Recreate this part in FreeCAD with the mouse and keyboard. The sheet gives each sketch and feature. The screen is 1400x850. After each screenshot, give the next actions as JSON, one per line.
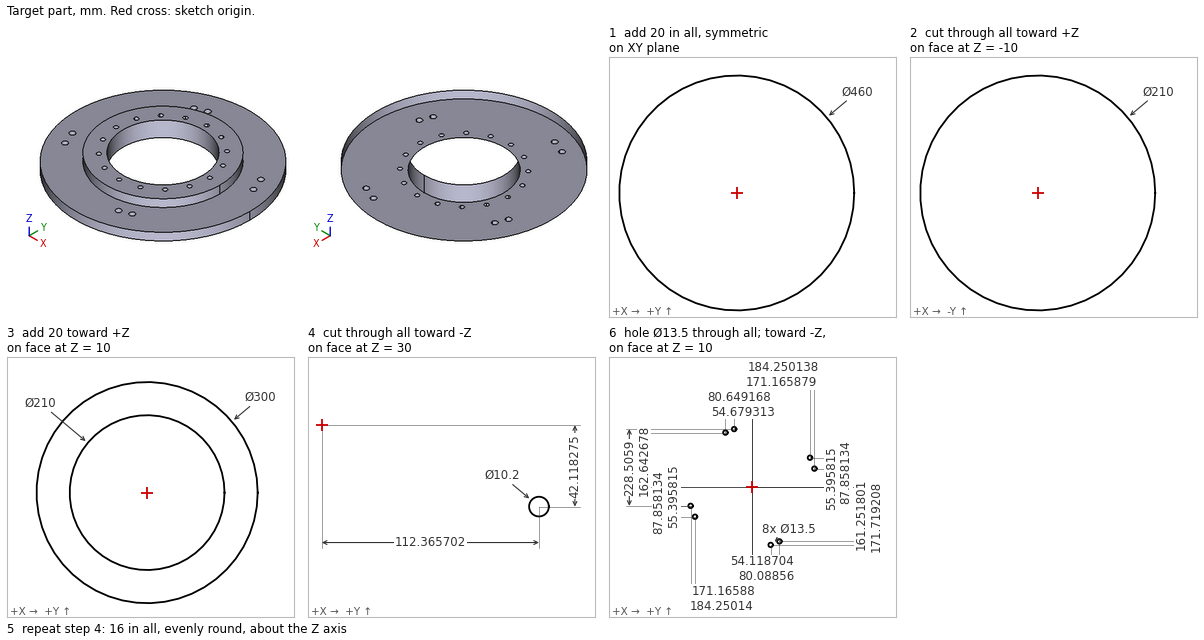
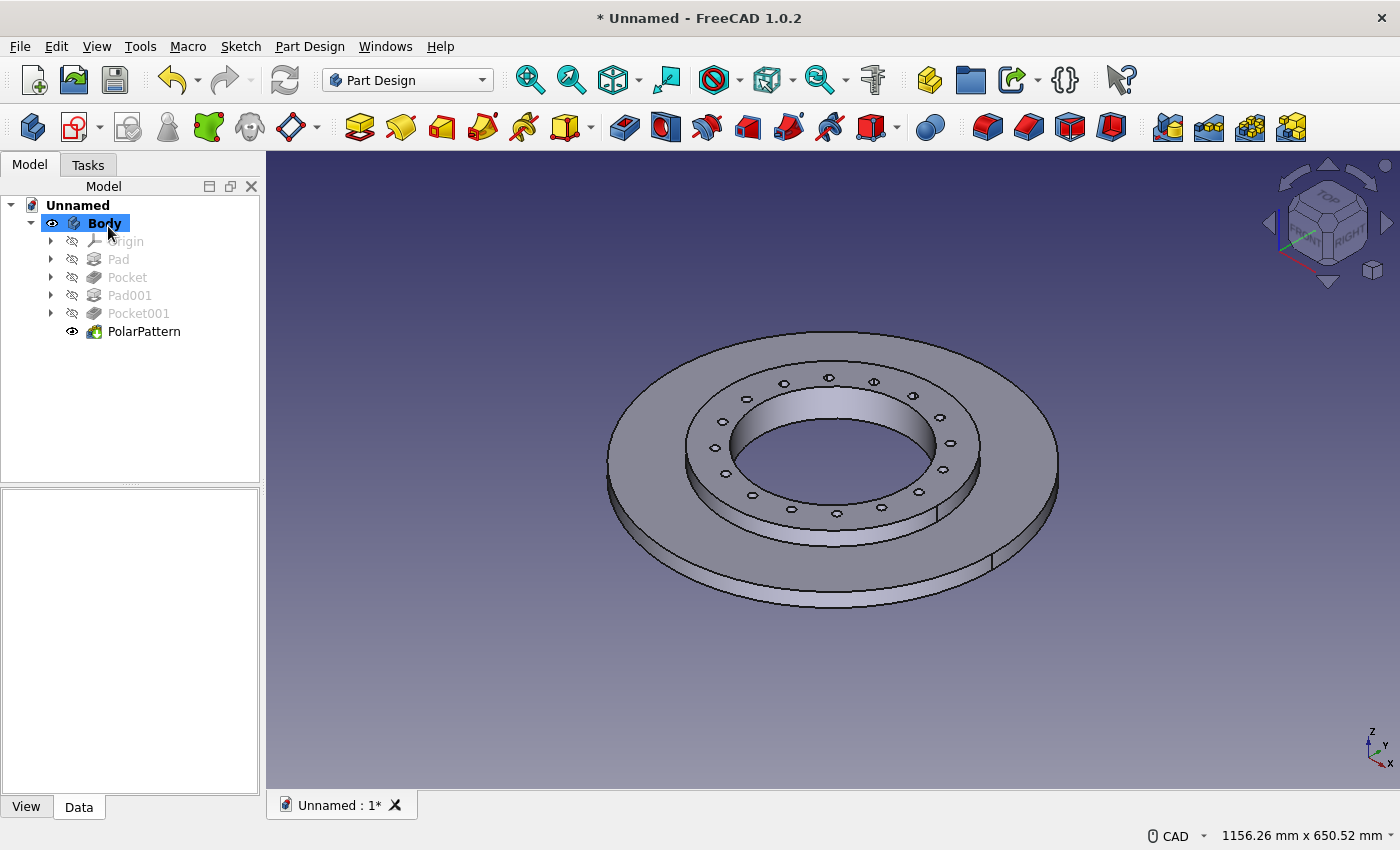
{"action": "left_click", "coordinate": [1015, 461]}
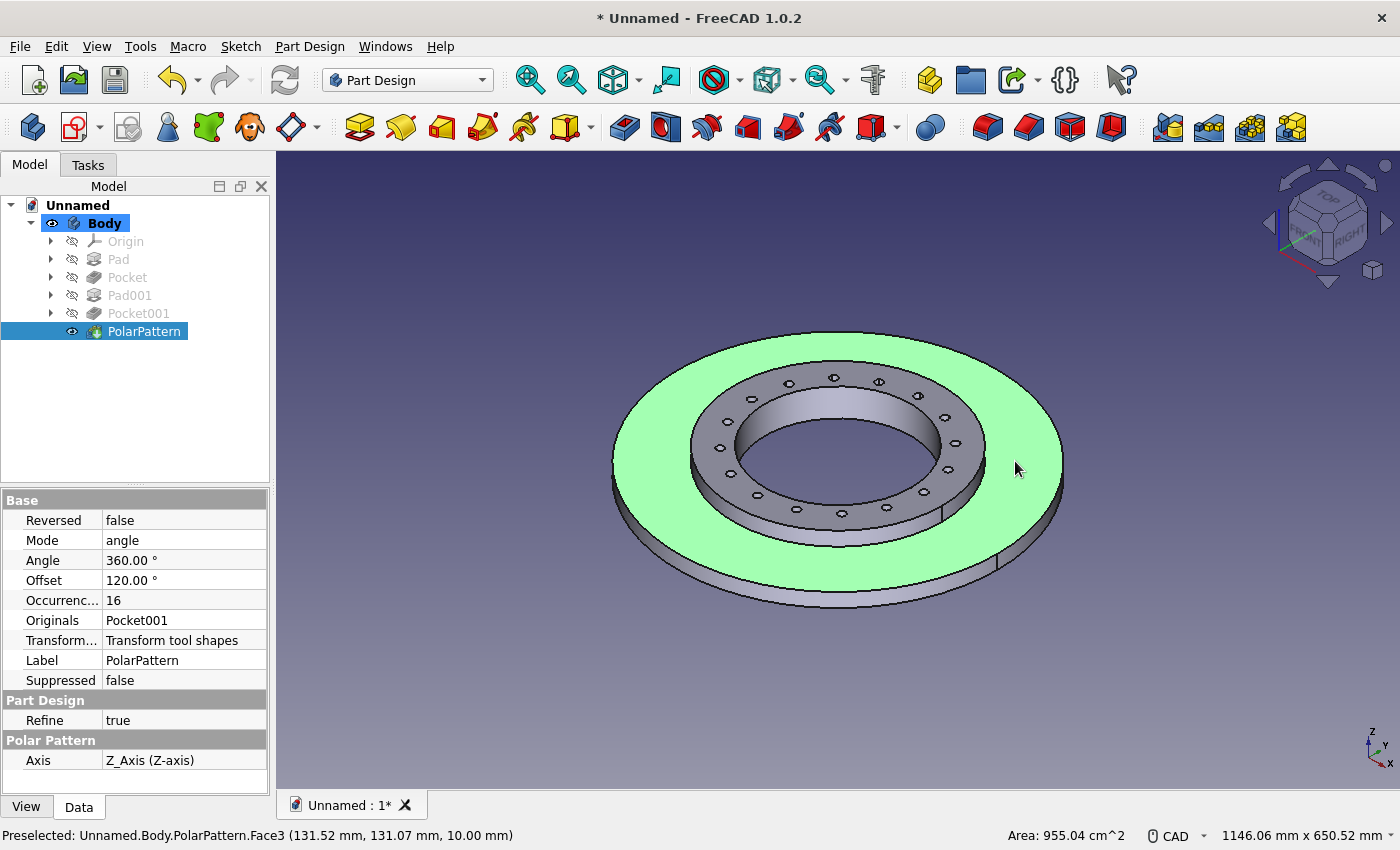
{"action": "left_click", "coordinate": [74, 128]}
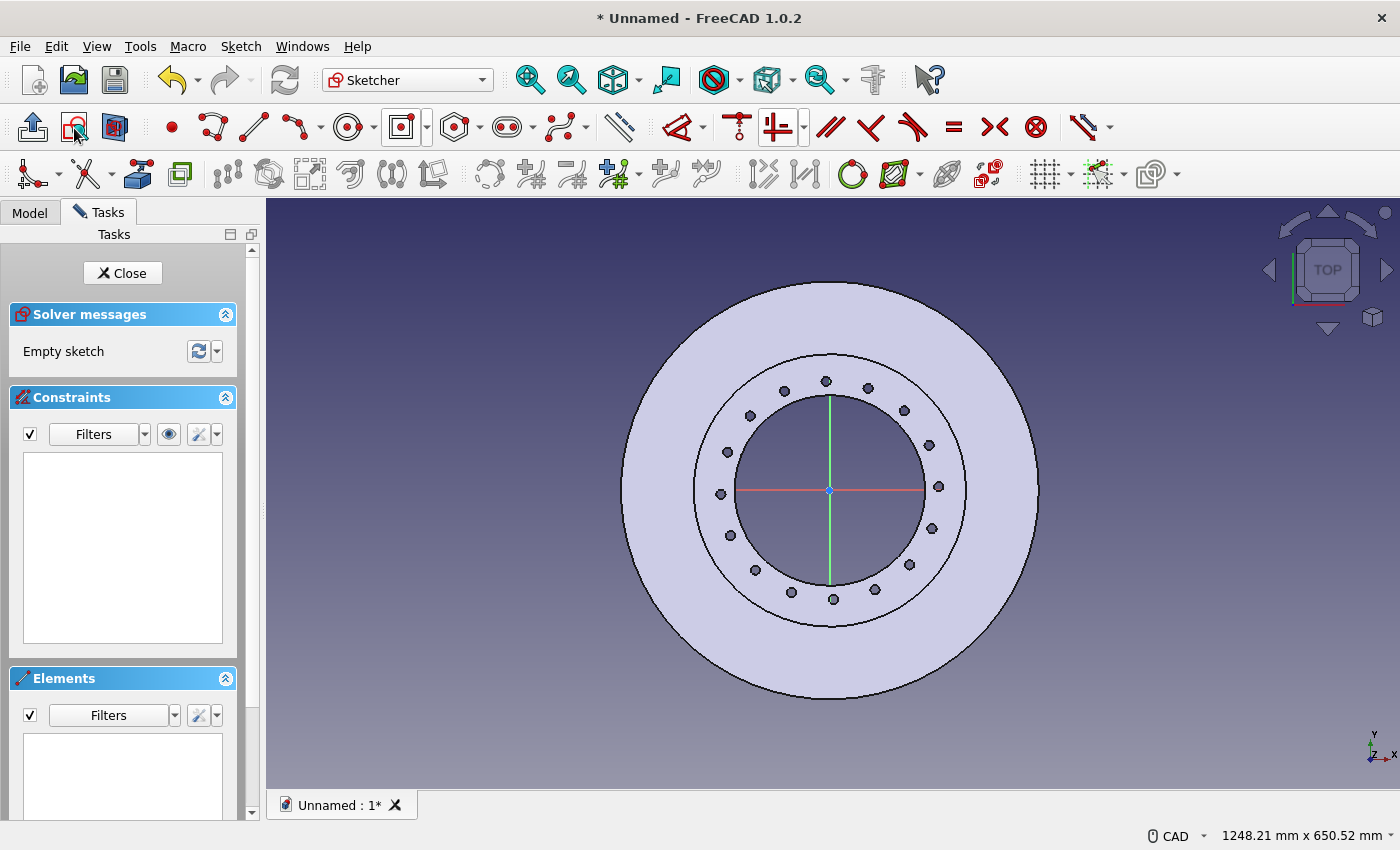
{"action": "key", "text": "g c"}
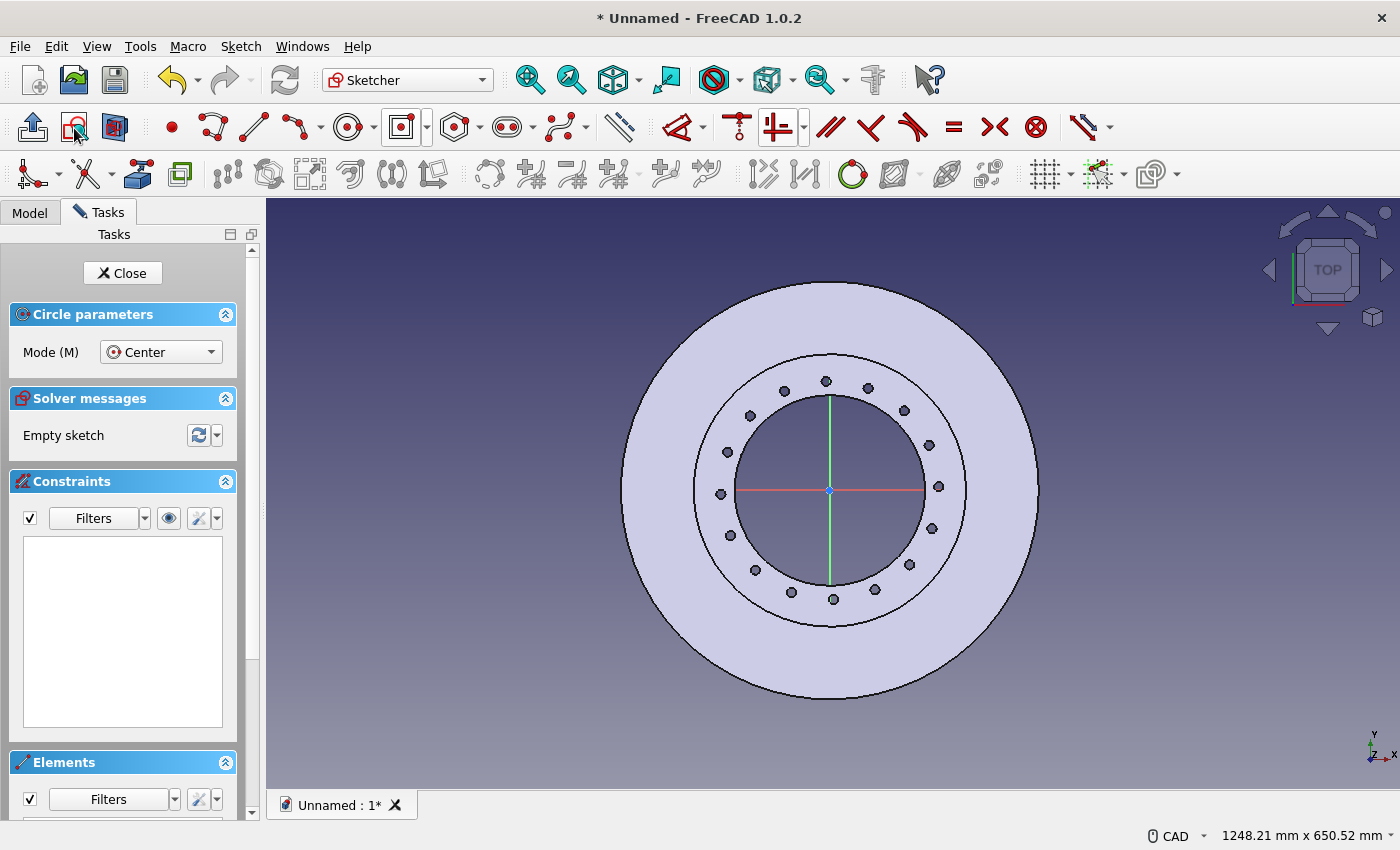
{"action": "scroll", "coordinate": [879, 646], "scroll_direction": "up", "scroll_amount": 7}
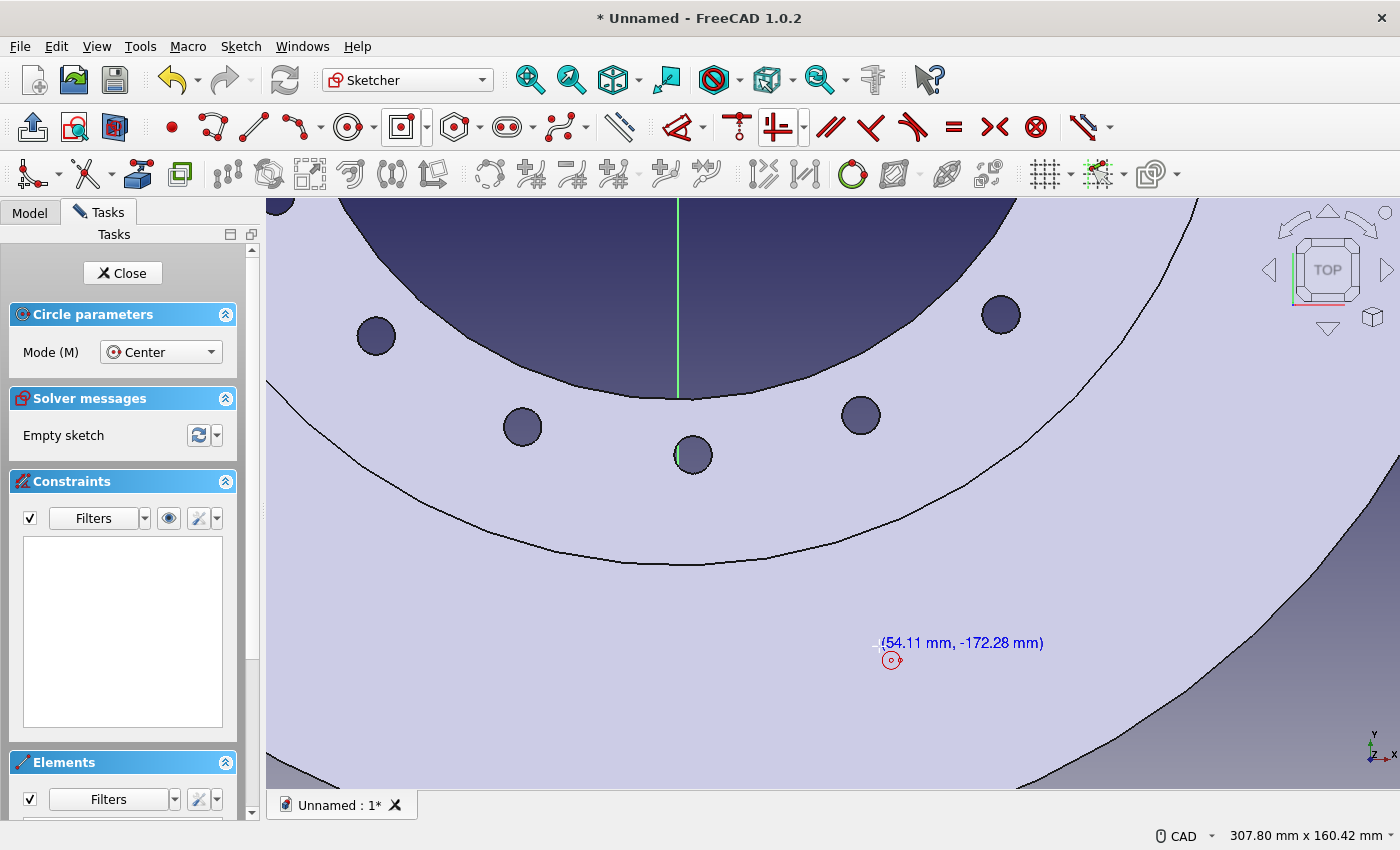
{"action": "scroll", "coordinate": [802, 702], "scroll_direction": "down", "scroll_amount": 6}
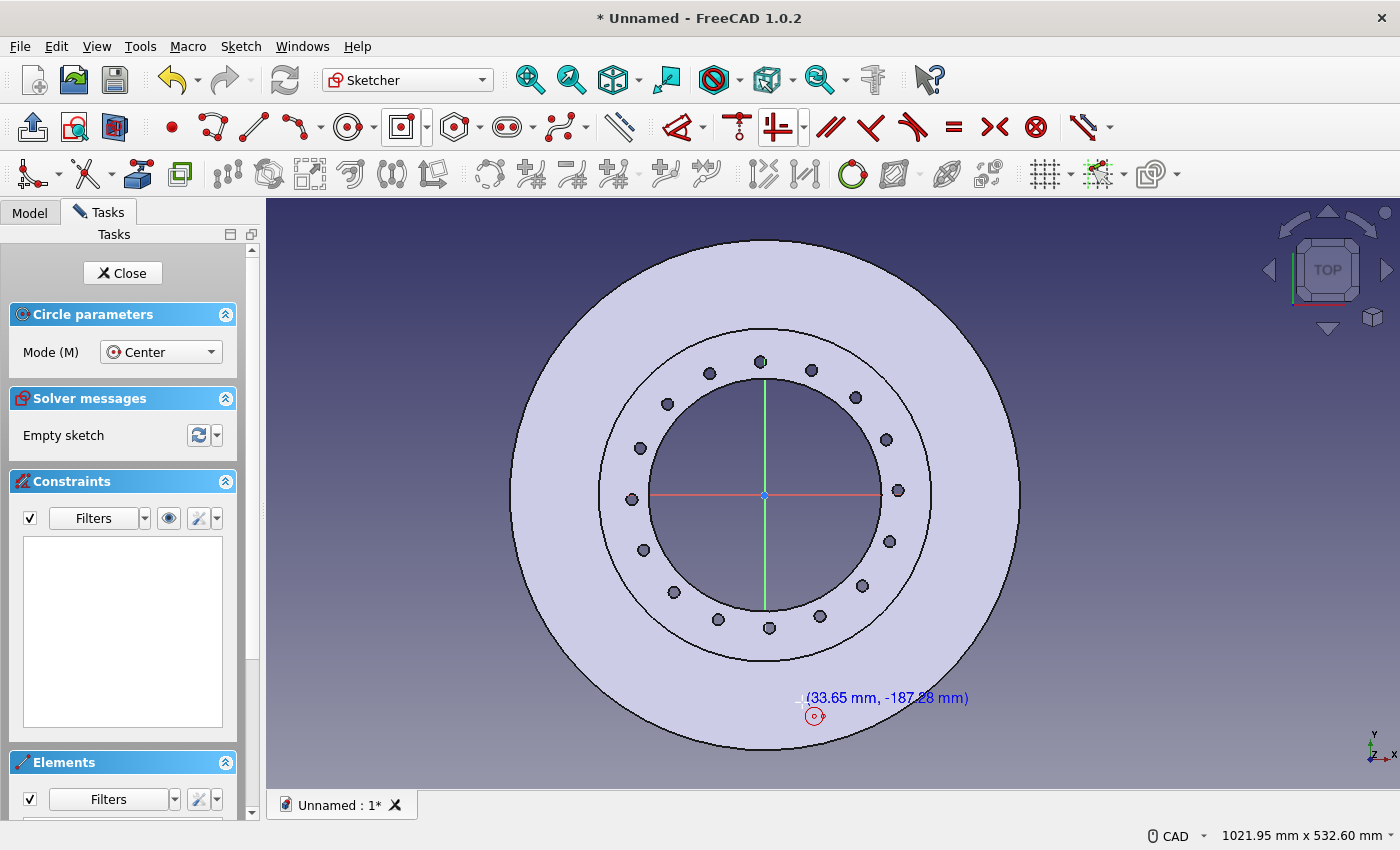
{"action": "left_click", "coordinate": [825, 686]}
{"action": "mouse_move", "coordinate": [830, 680]}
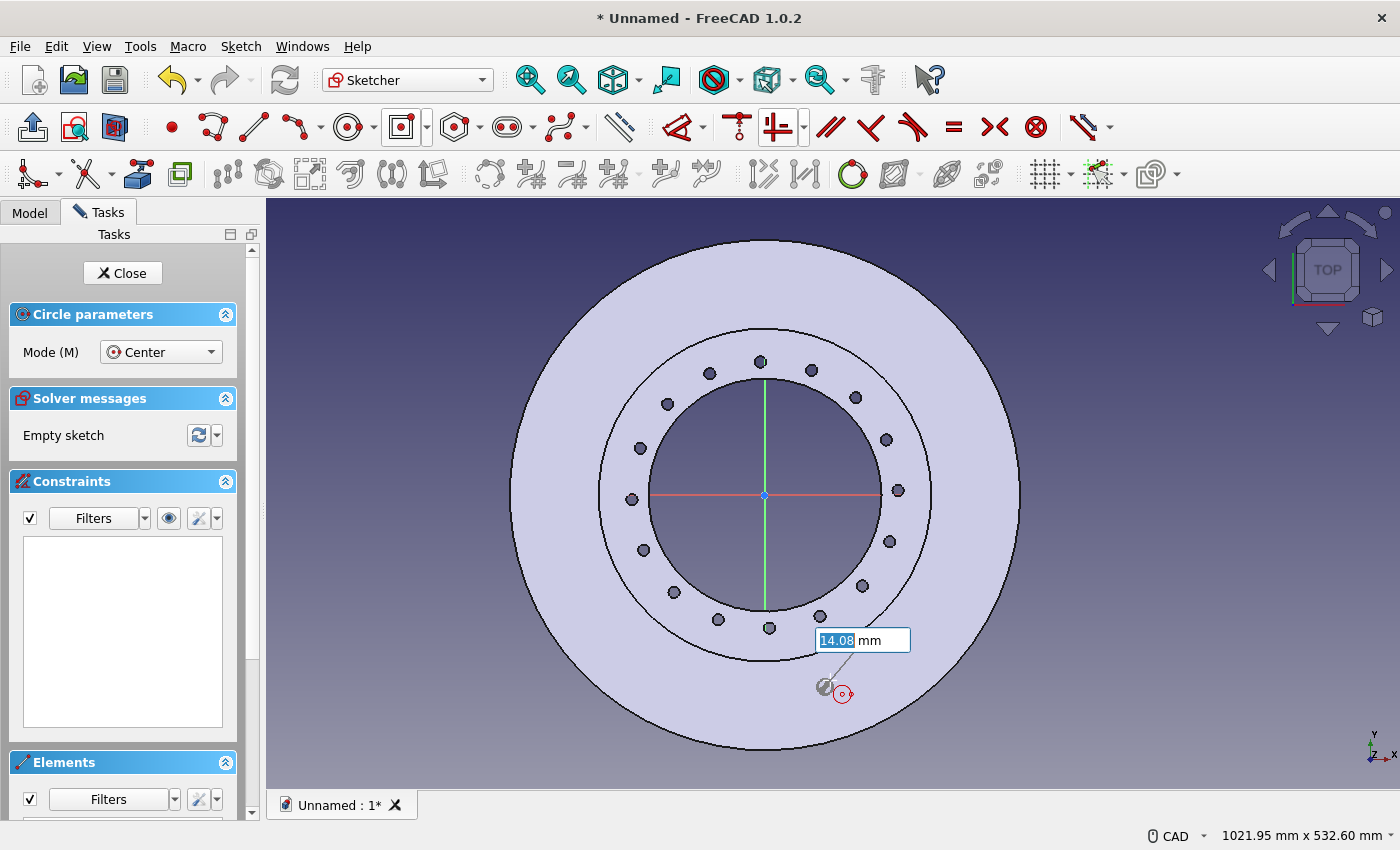
{"action": "type", "text": "13.5"}
{"action": "key", "text": "Return"}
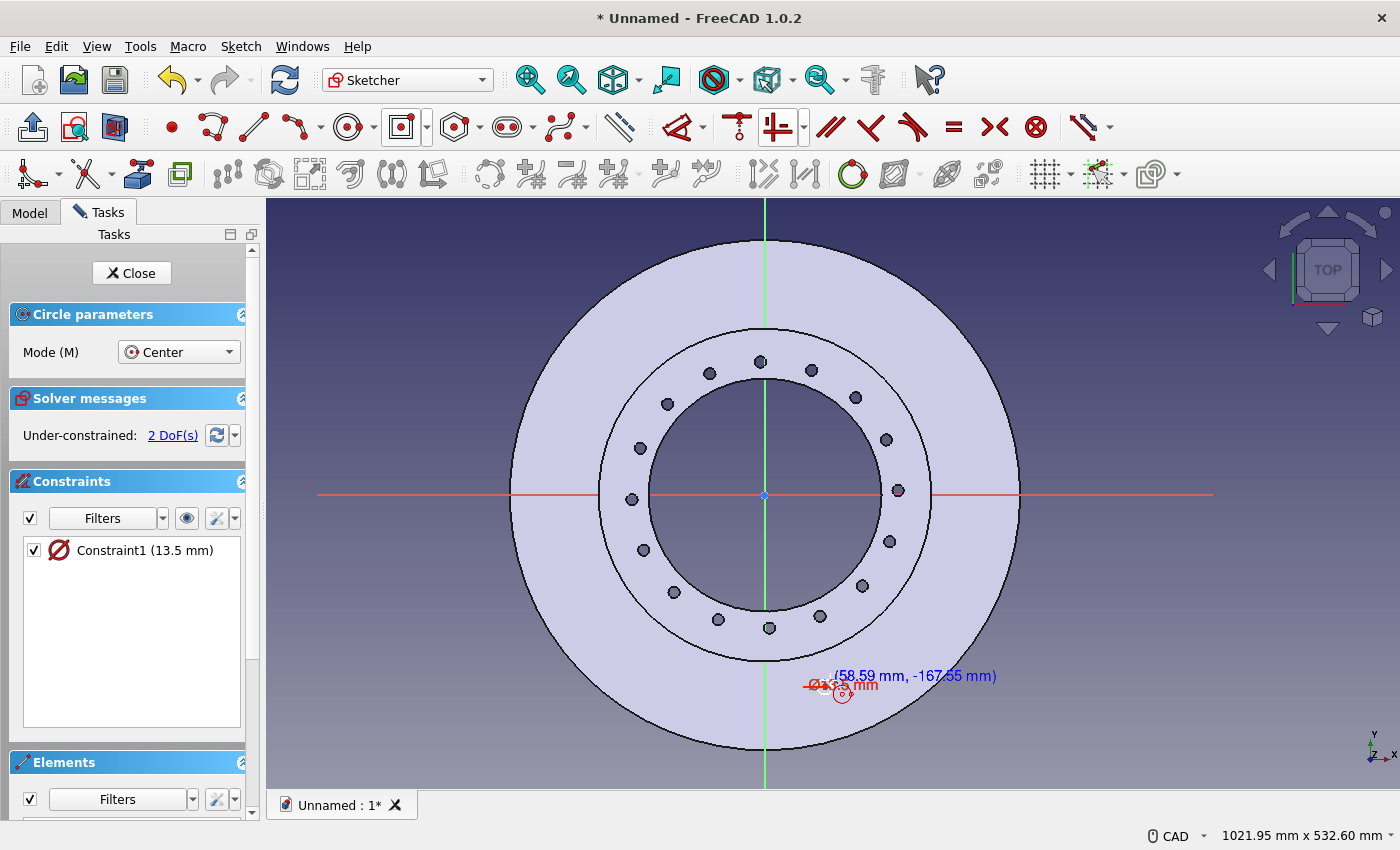
{"action": "scroll", "coordinate": [854, 674], "scroll_direction": "up", "scroll_amount": 6}